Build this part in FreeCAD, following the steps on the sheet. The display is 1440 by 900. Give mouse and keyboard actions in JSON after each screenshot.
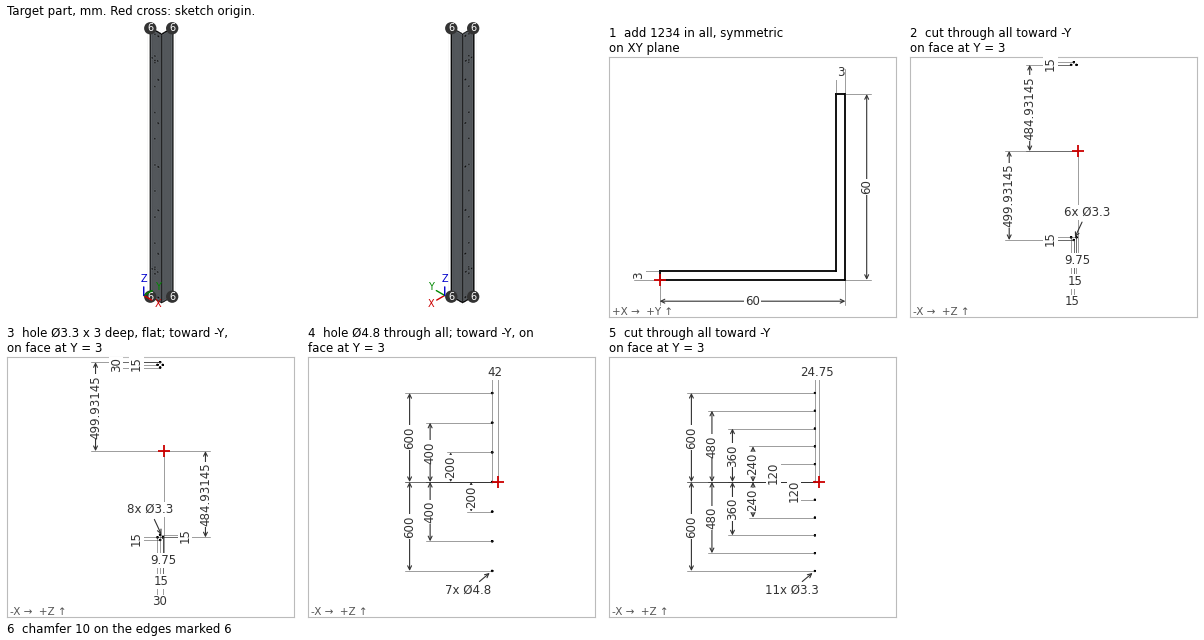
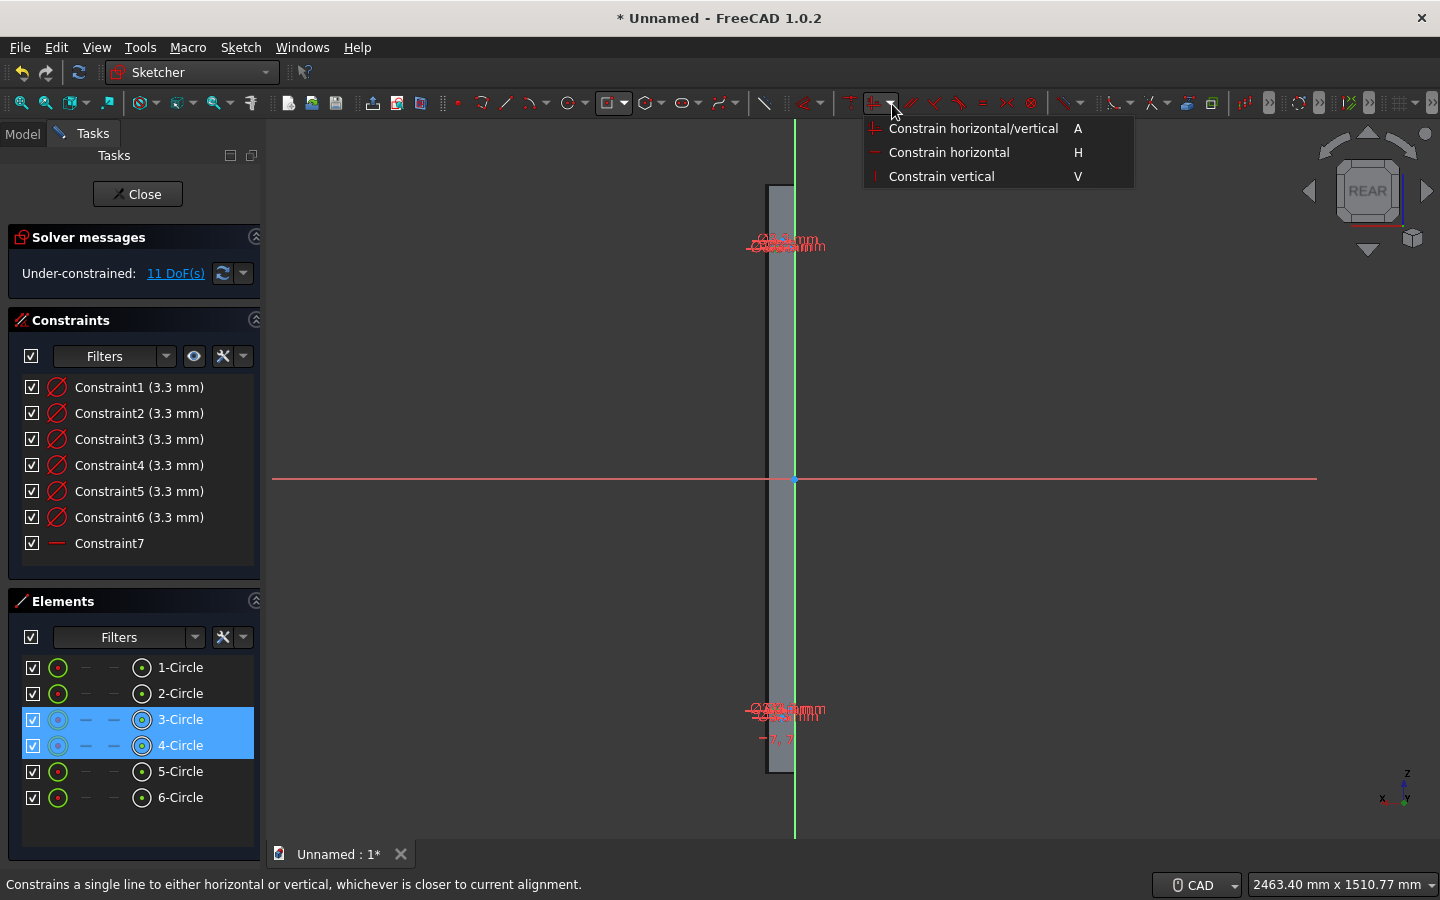
{"action": "left_click", "coordinate": [999, 176]}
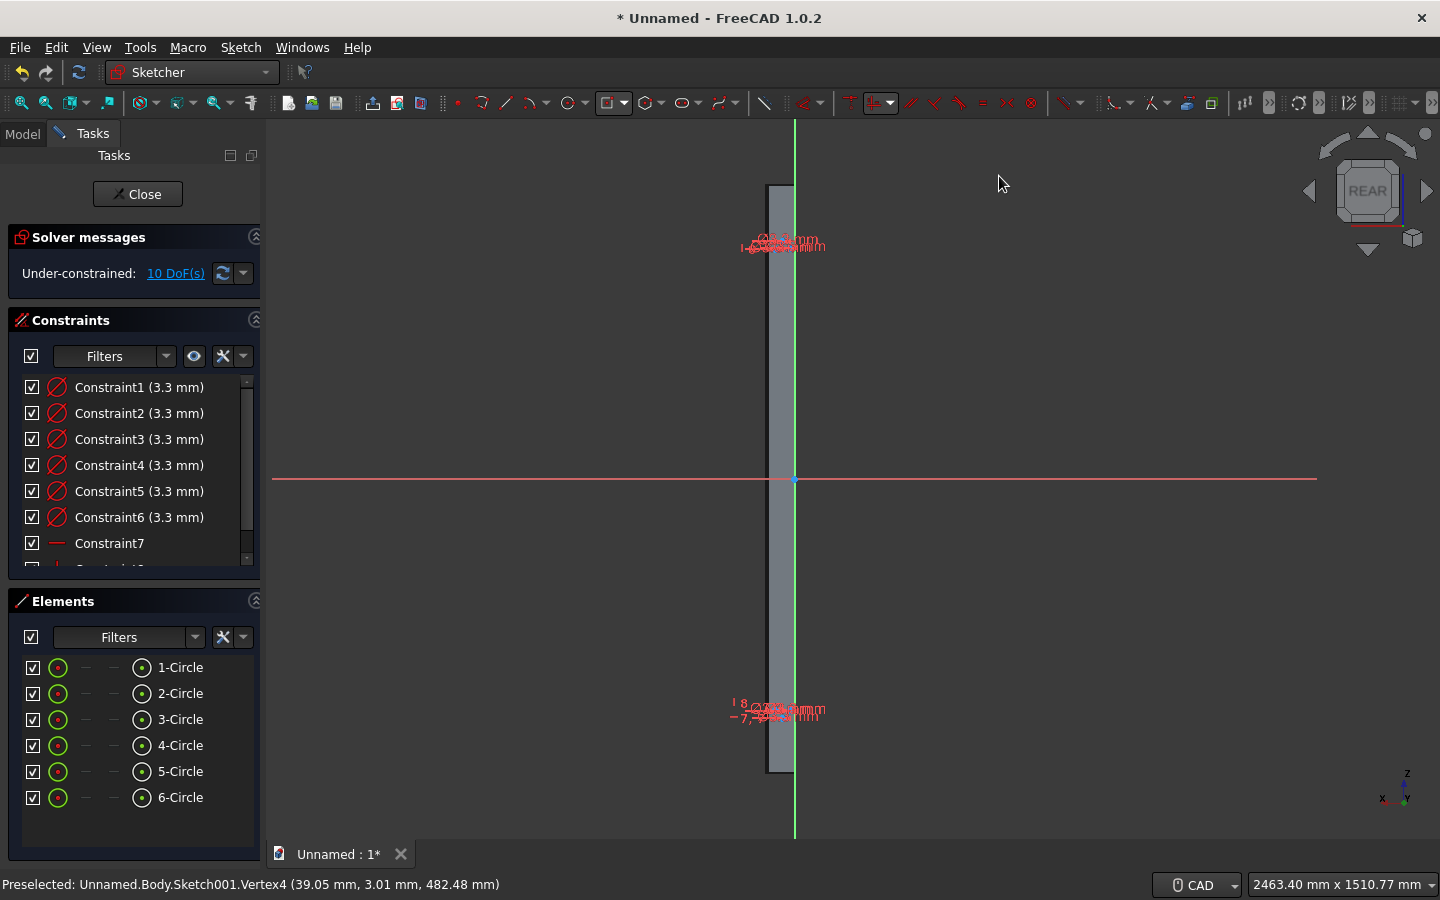
{"action": "left_click", "coordinate": [790, 711]}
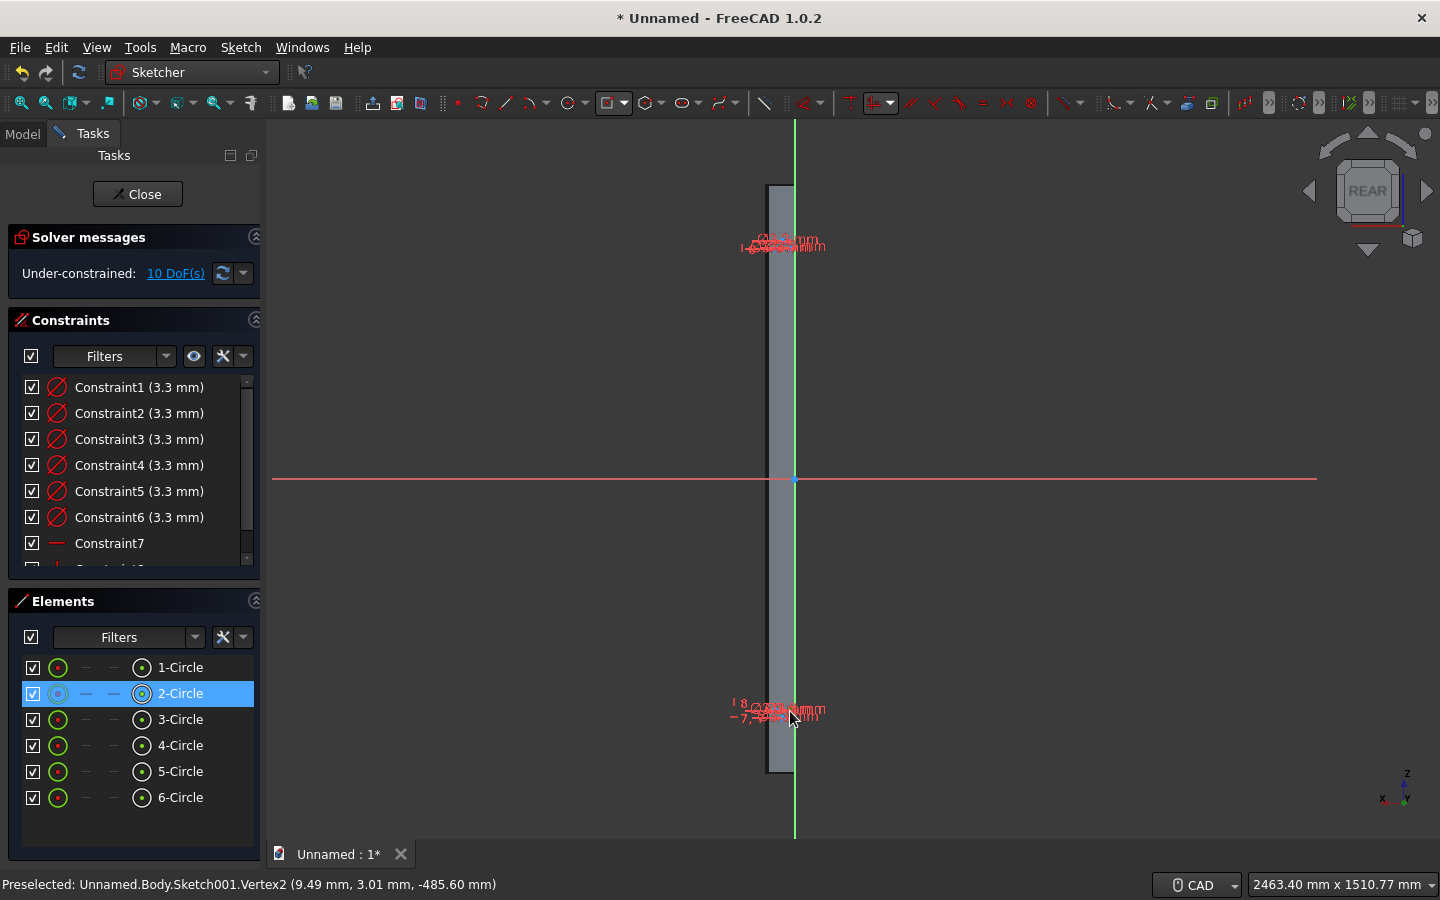
{"action": "left_click", "coordinate": [790, 248]}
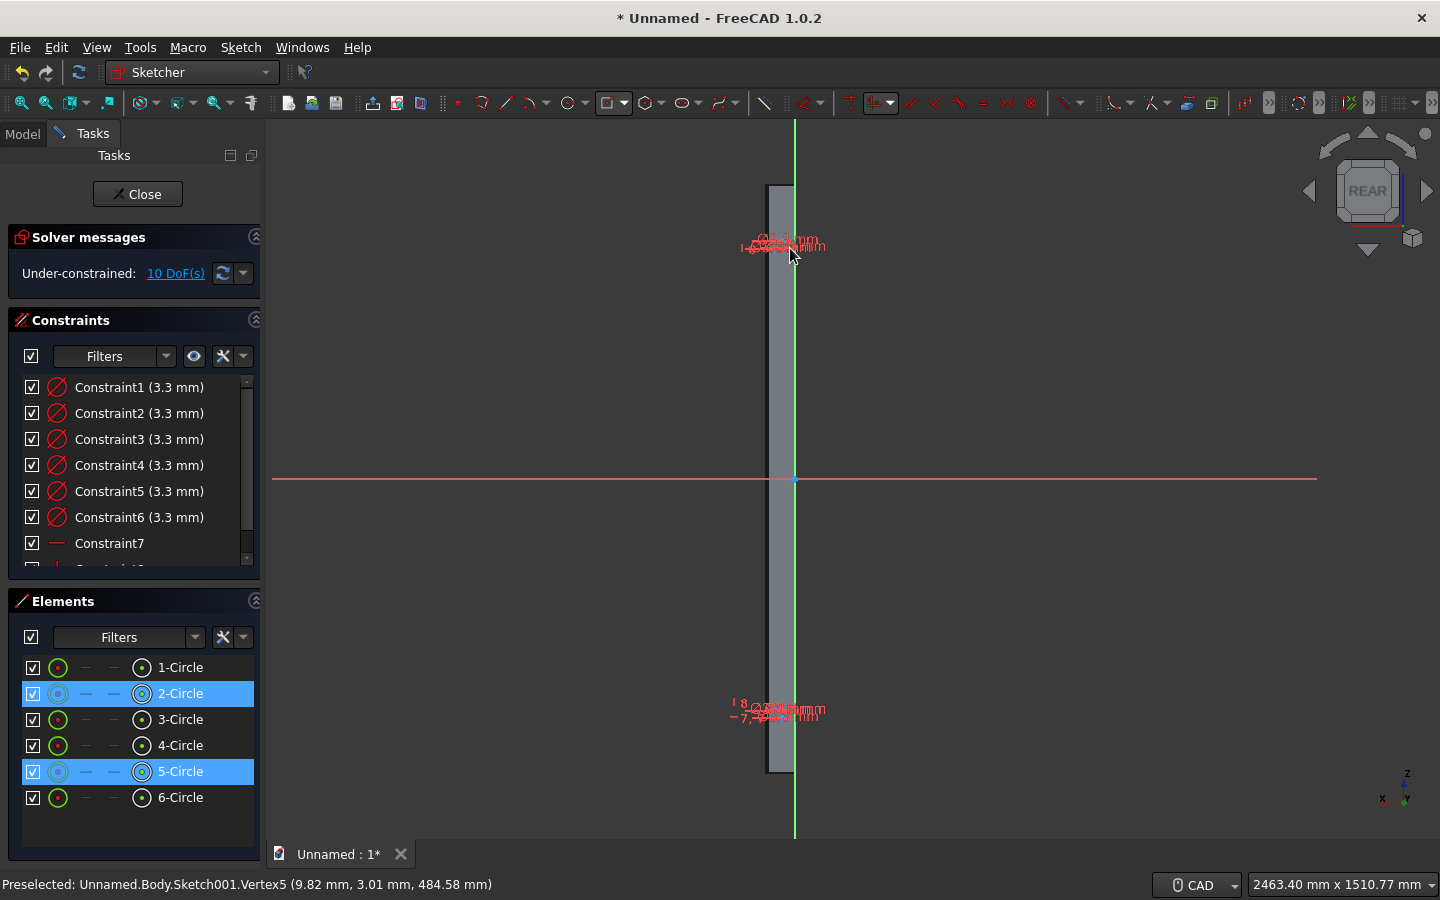
{"action": "left_click", "coordinate": [892, 104]}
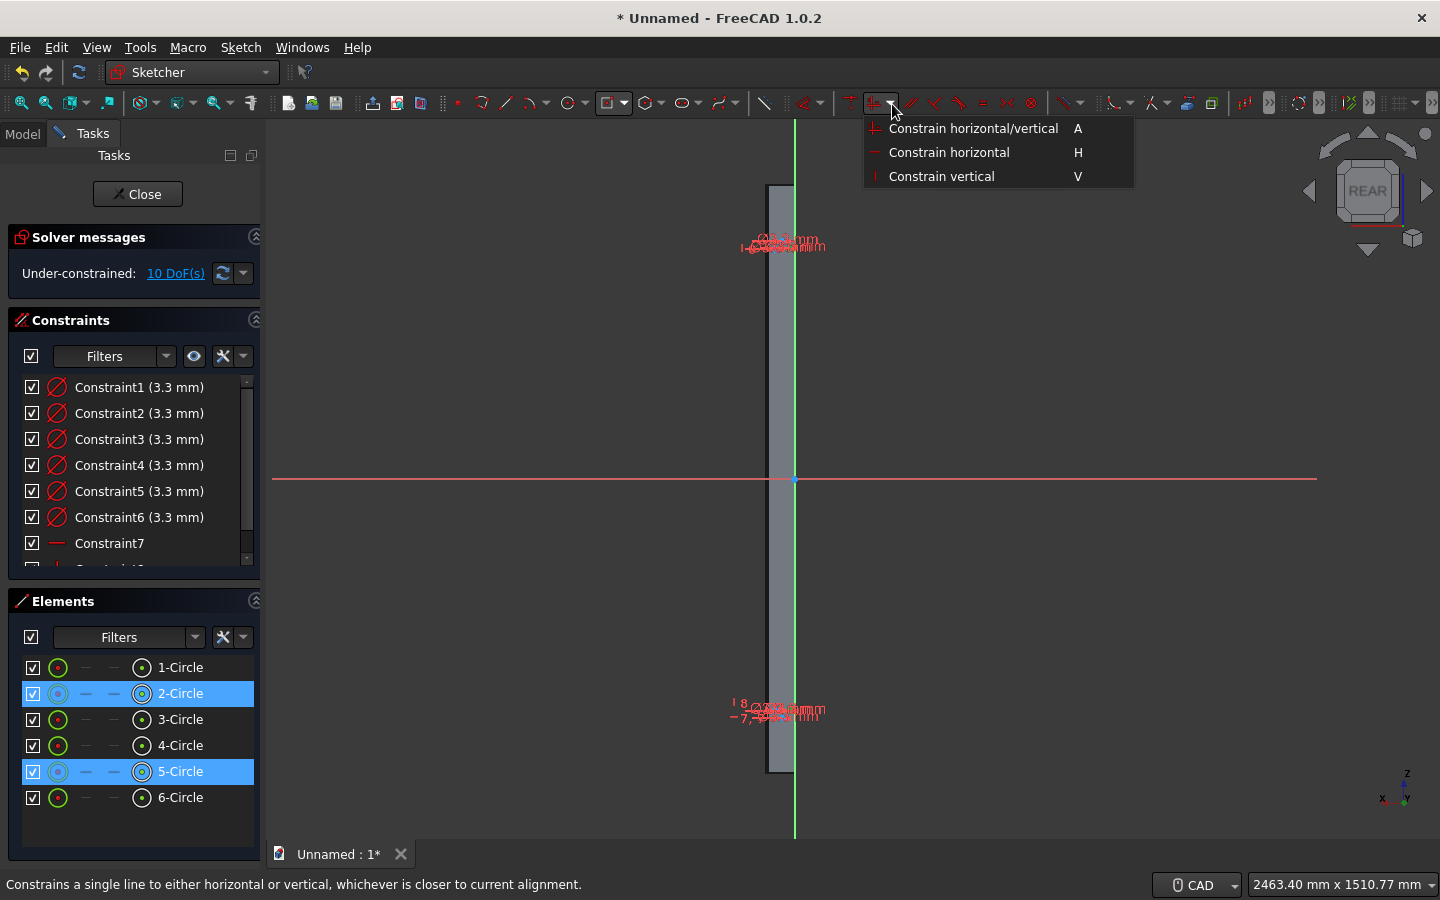
{"action": "left_click", "coordinate": [999, 176]}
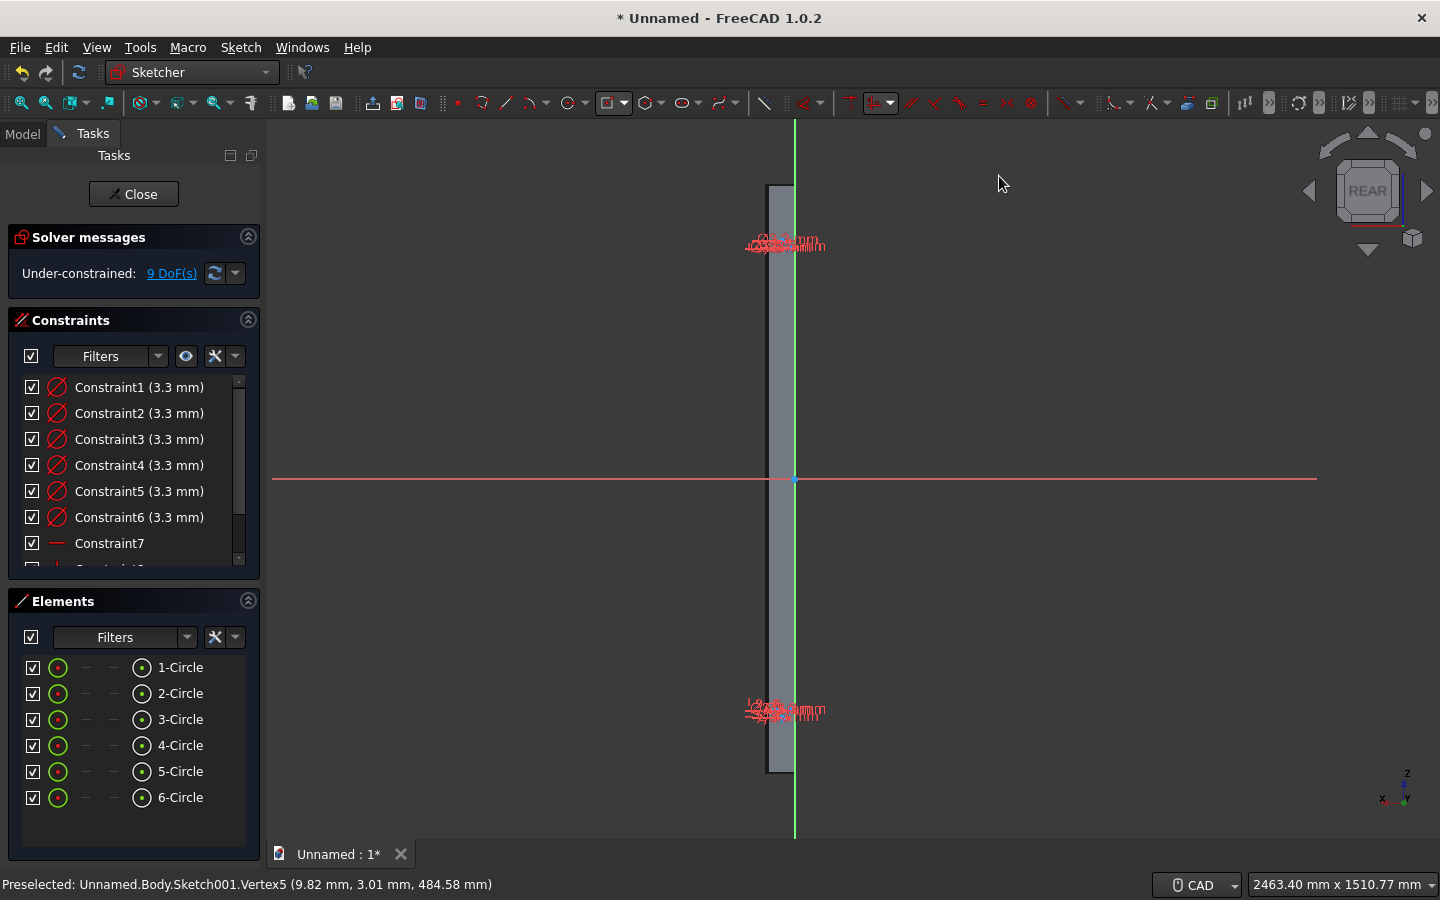
{"action": "scroll", "coordinate": [776, 249], "scroll_direction": "up", "scroll_amount": 4}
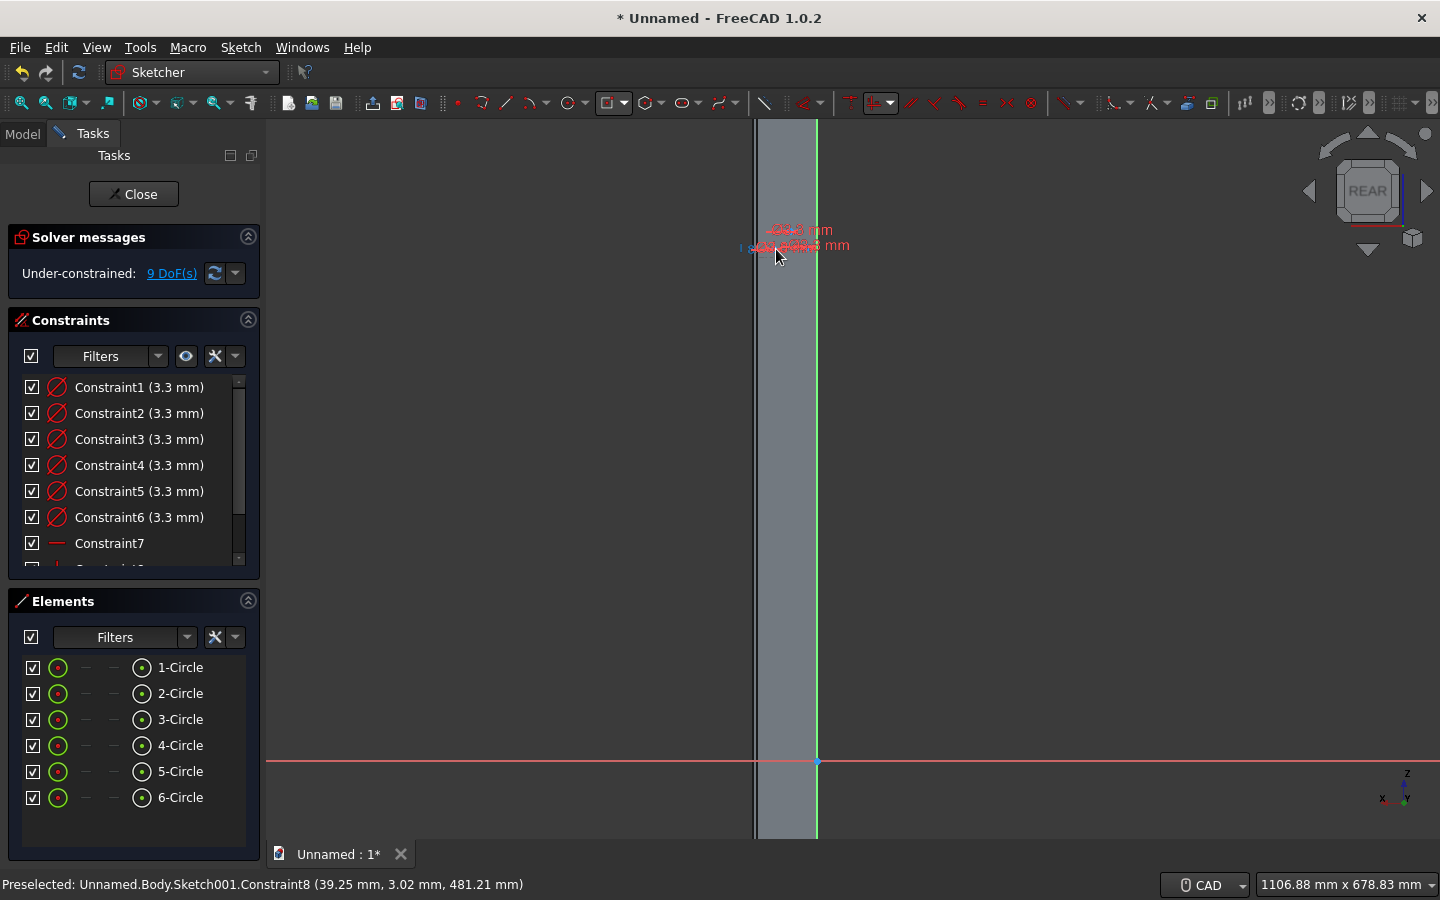
{"action": "scroll", "coordinate": [774, 250], "scroll_direction": "up", "scroll_amount": 4}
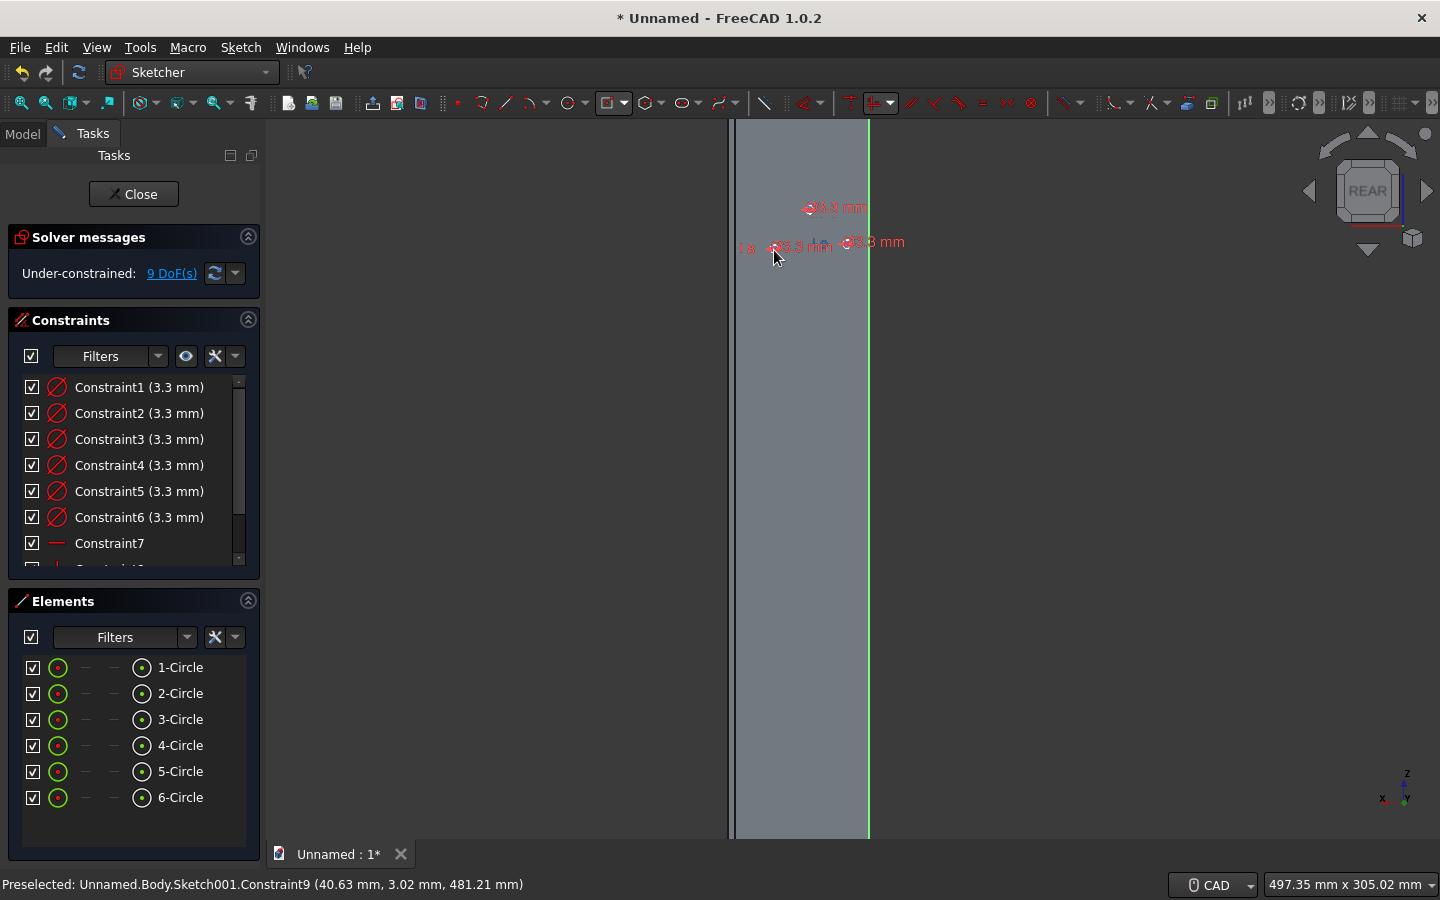
{"action": "left_click", "coordinate": [774, 249]}